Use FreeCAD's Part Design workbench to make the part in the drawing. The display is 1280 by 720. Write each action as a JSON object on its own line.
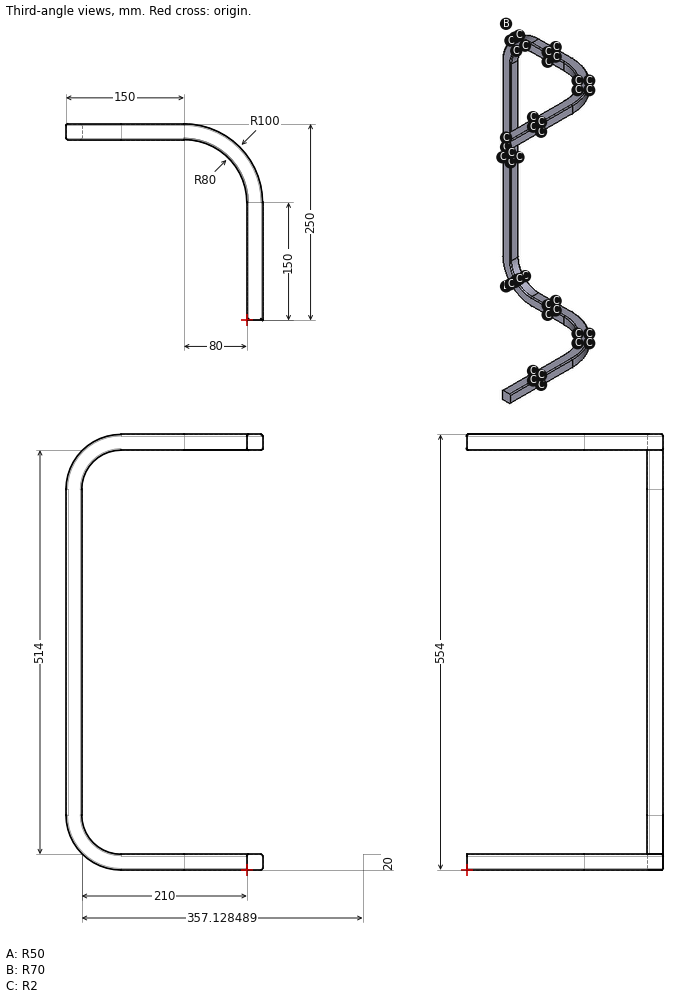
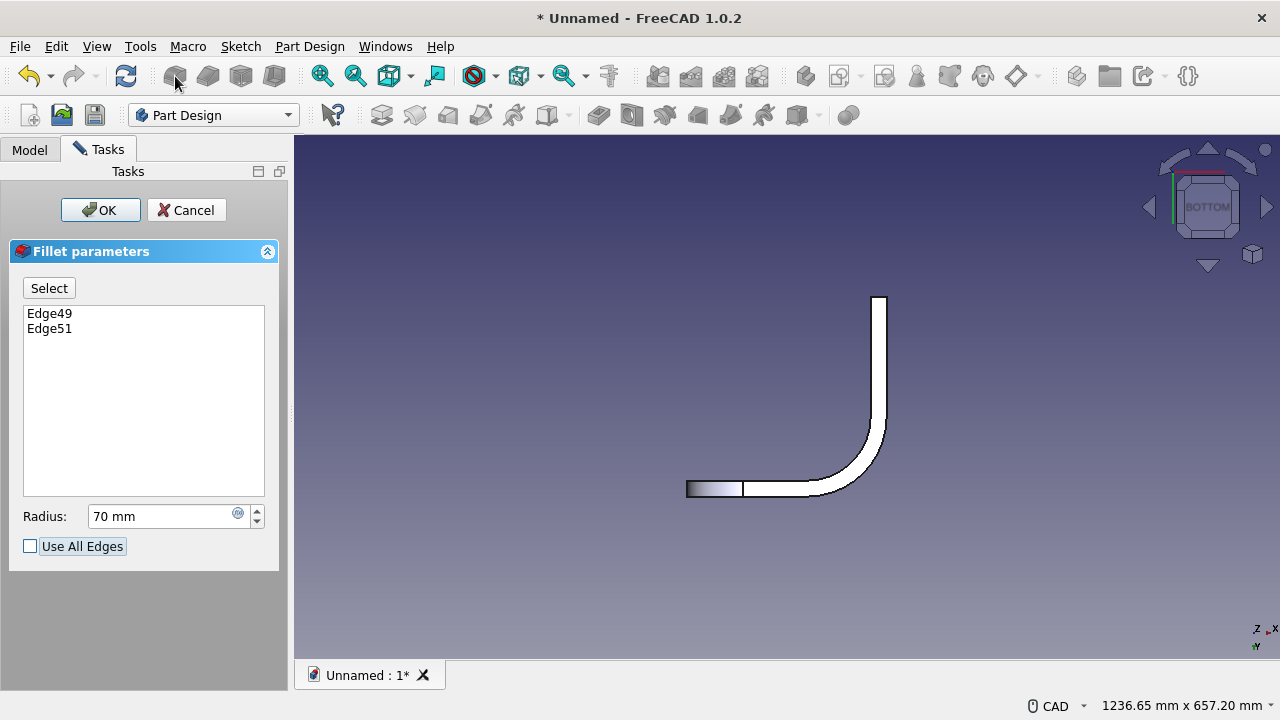
{"action": "left_click", "coordinate": [101, 210]}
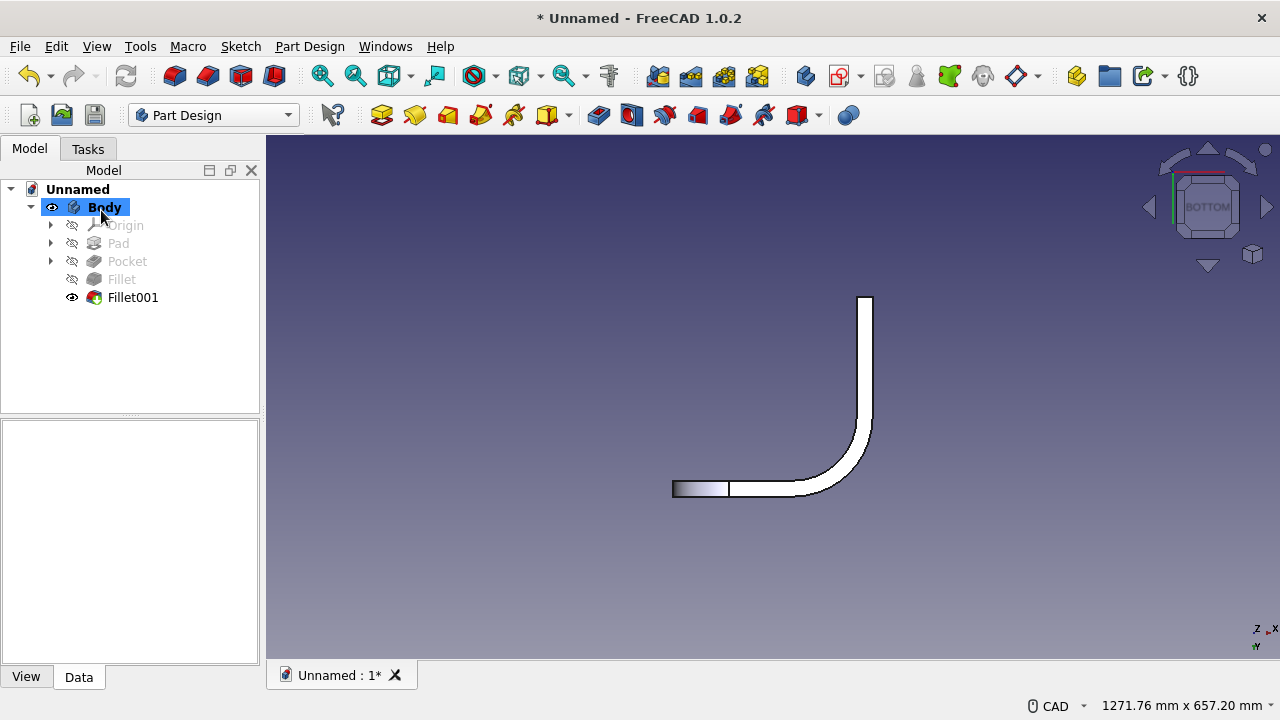
{"action": "left_click", "coordinate": [323, 76]}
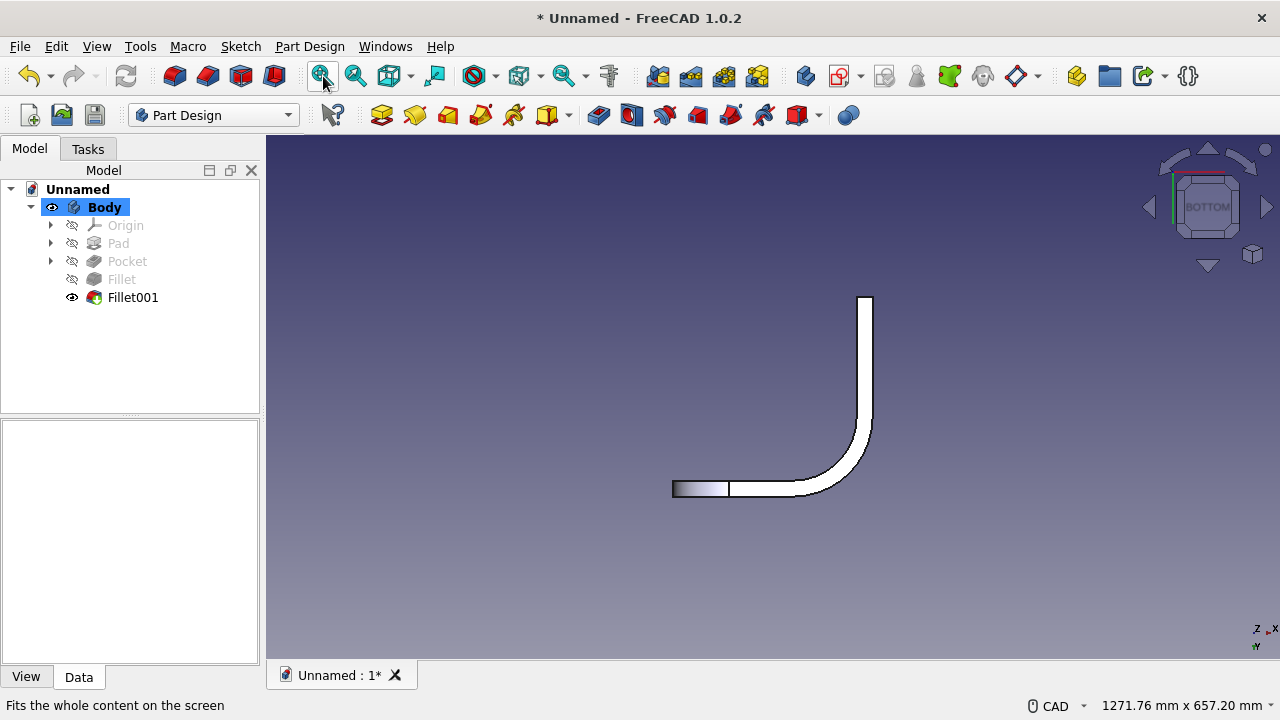
{"action": "left_click", "coordinate": [873, 356]}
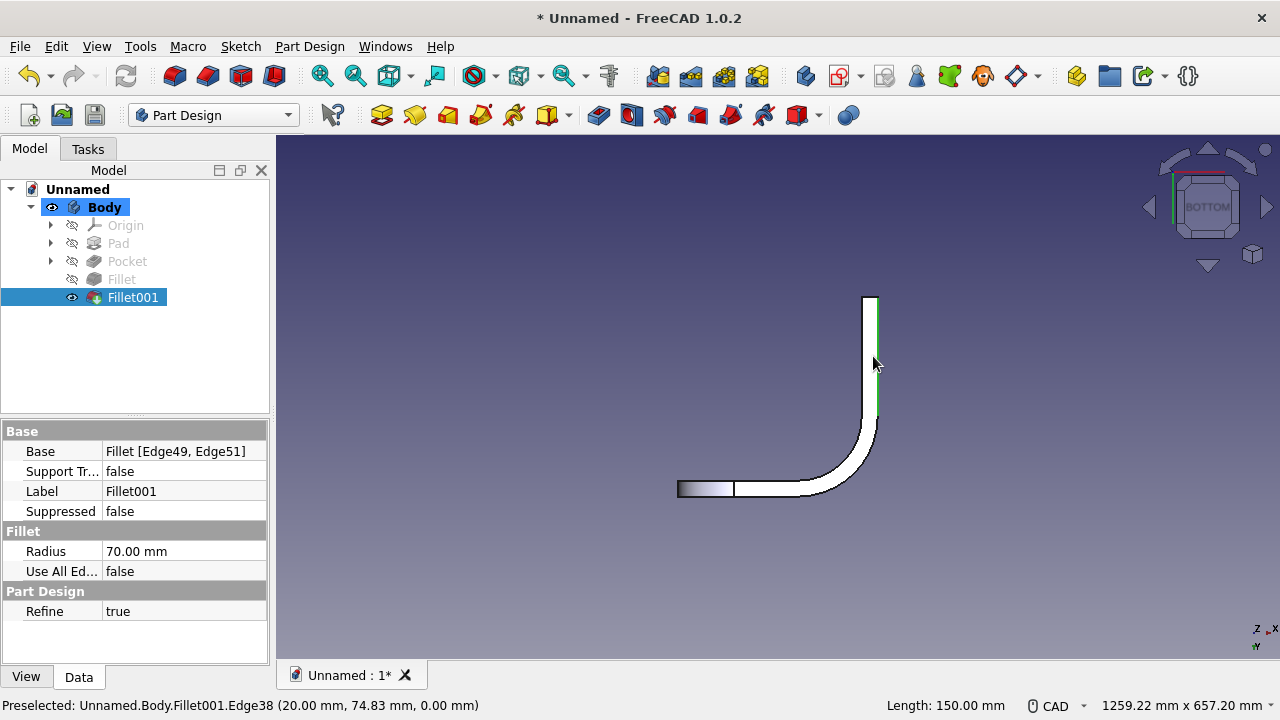
{"action": "left_click", "coordinate": [766, 480], "text": "ctrl"}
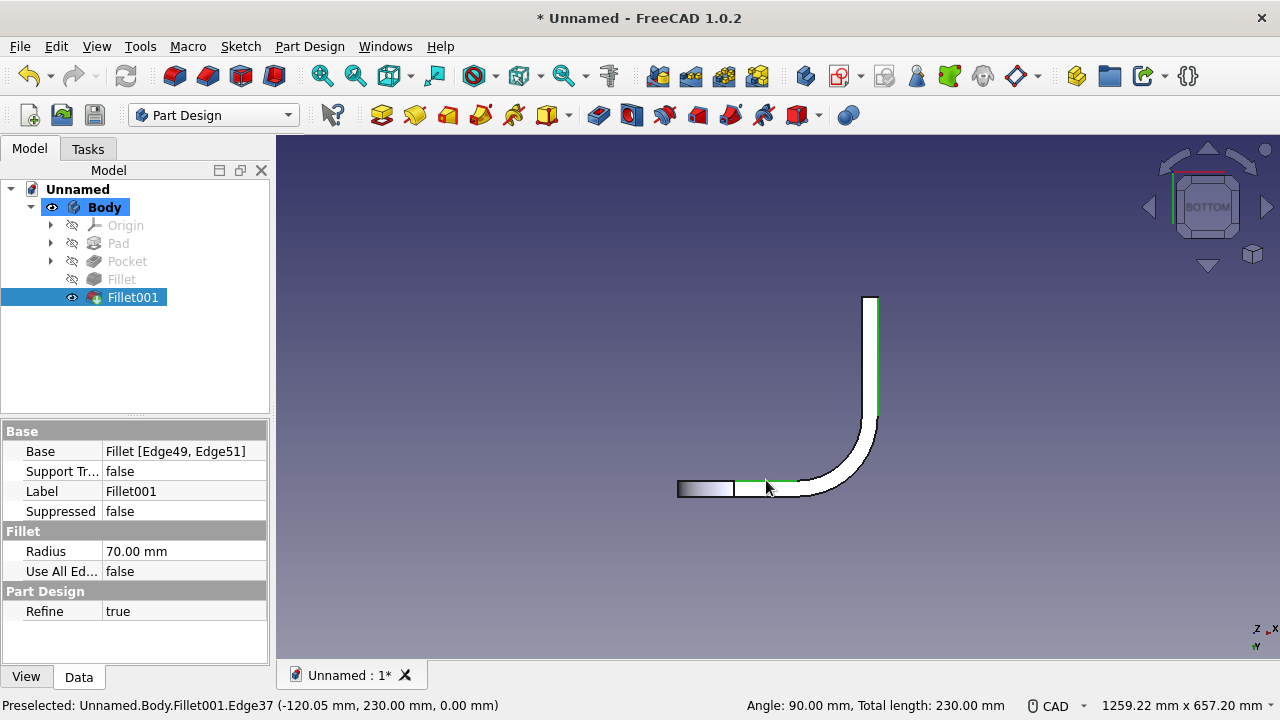
{"action": "left_click", "coordinate": [695, 480], "text": "ctrl"}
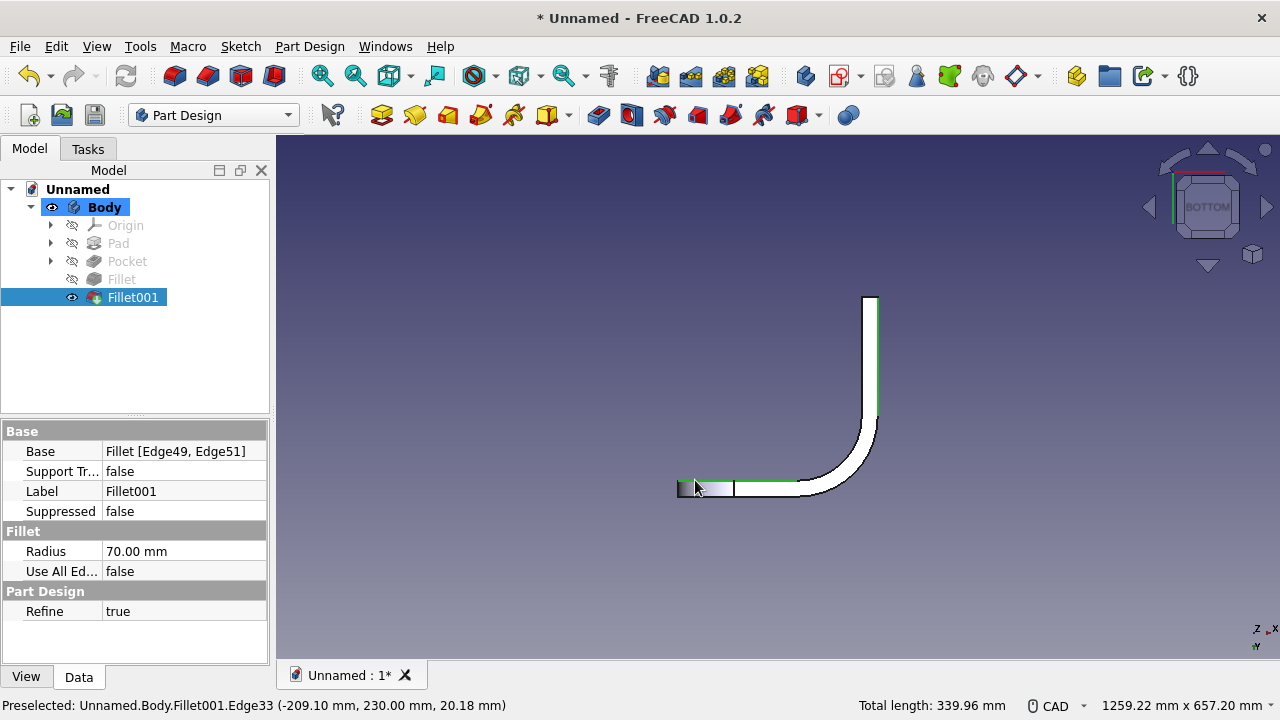
{"action": "left_click", "coordinate": [695, 496], "text": "ctrl"}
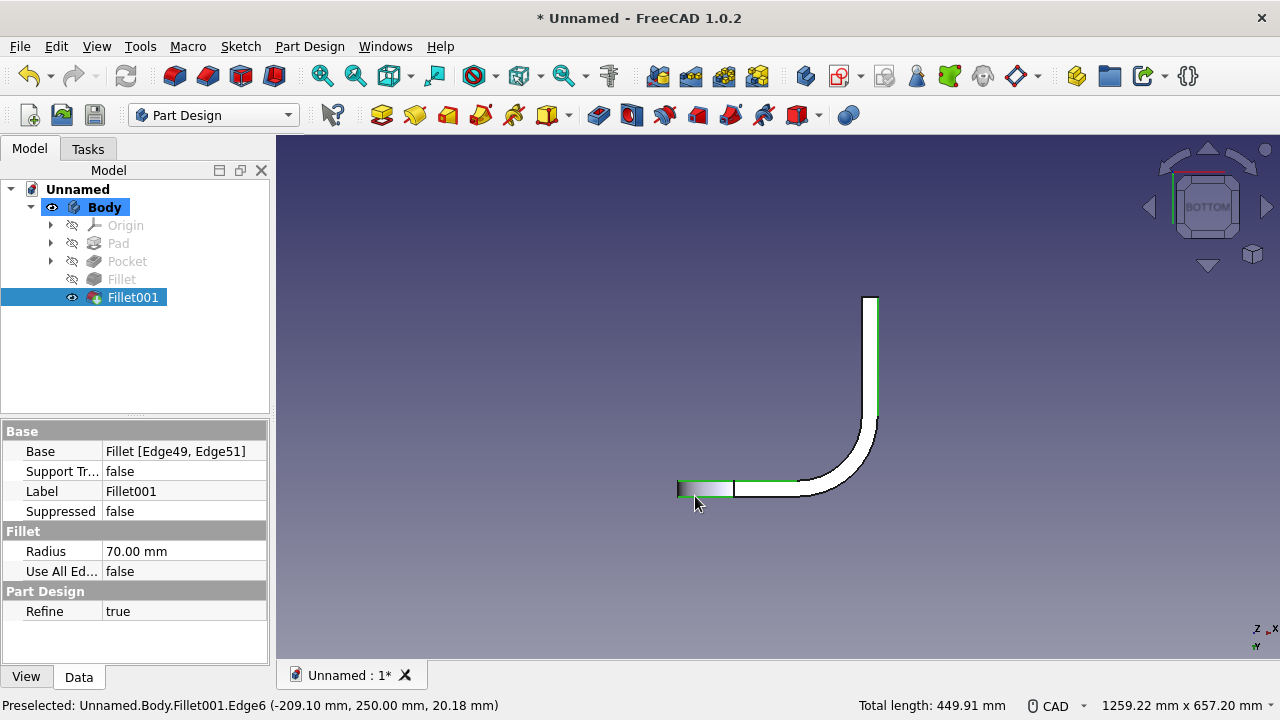
{"action": "left_click", "coordinate": [862, 356], "text": "ctrl"}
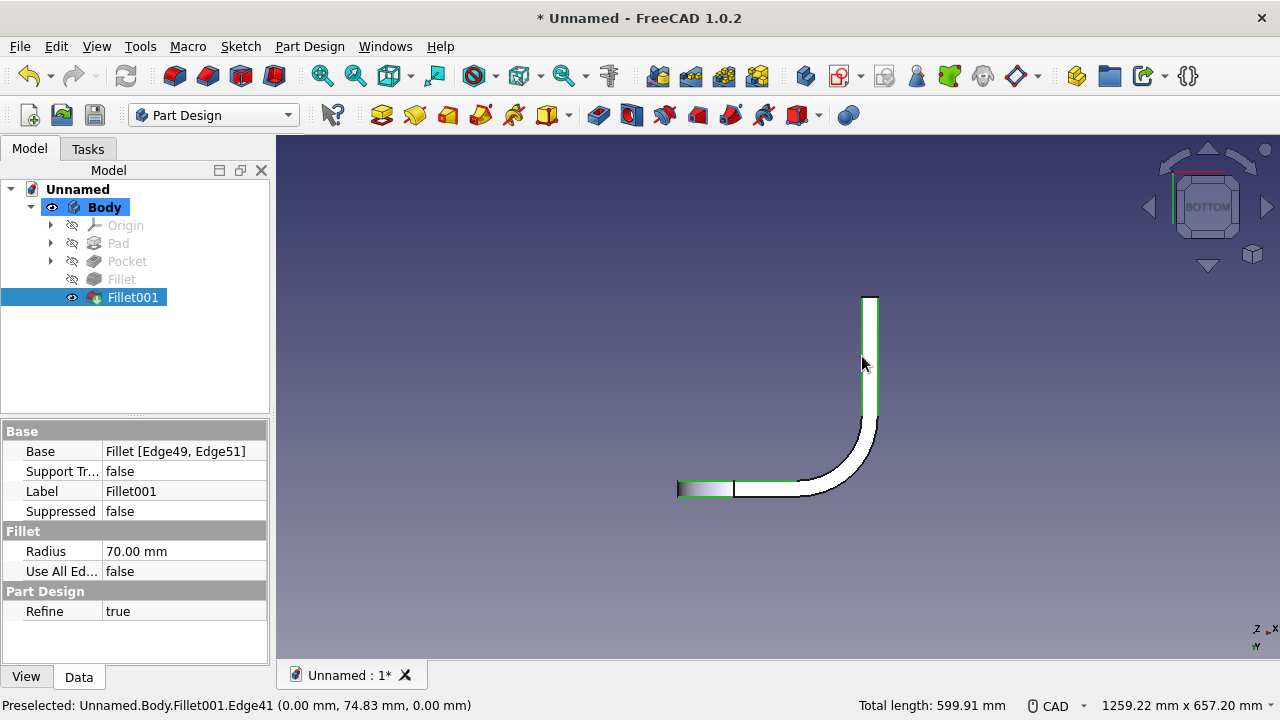
{"action": "left_click", "coordinate": [843, 461], "text": "ctrl"}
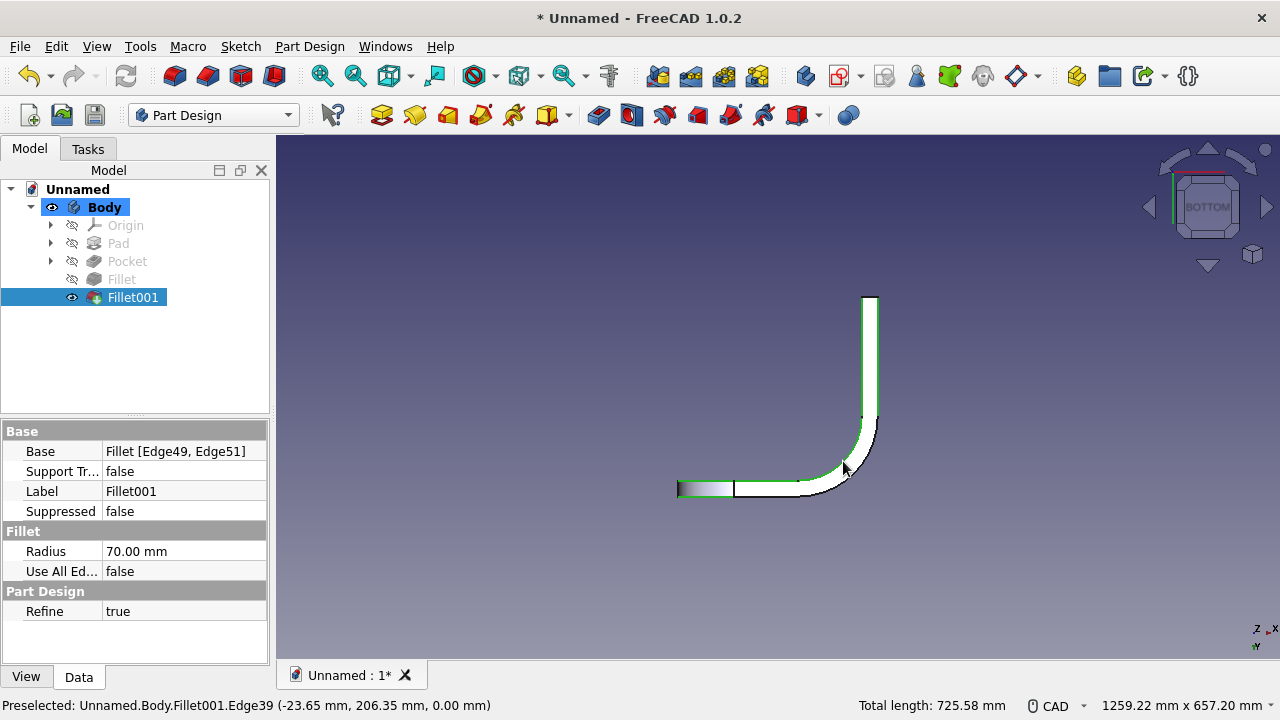
{"action": "left_click", "coordinate": [766, 496], "text": "ctrl"}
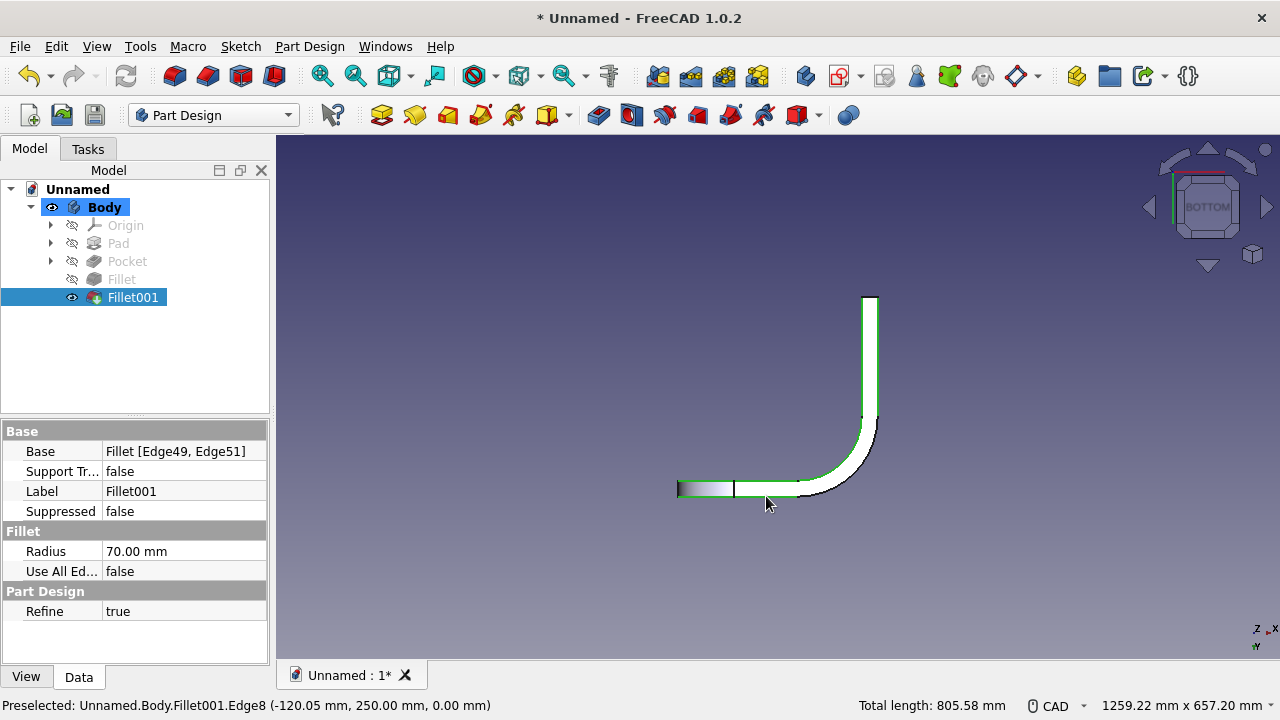
{"action": "left_click", "coordinate": [854, 472], "text": "ctrl"}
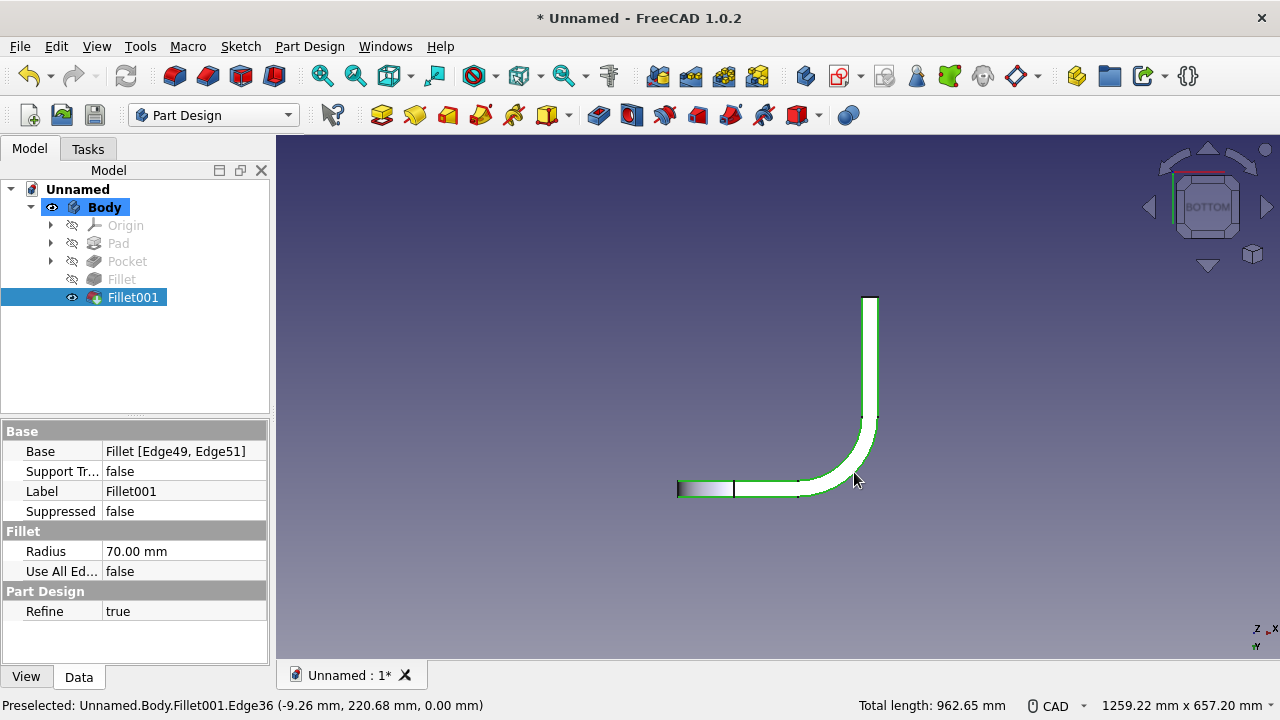
{"action": "key", "text": "0"}